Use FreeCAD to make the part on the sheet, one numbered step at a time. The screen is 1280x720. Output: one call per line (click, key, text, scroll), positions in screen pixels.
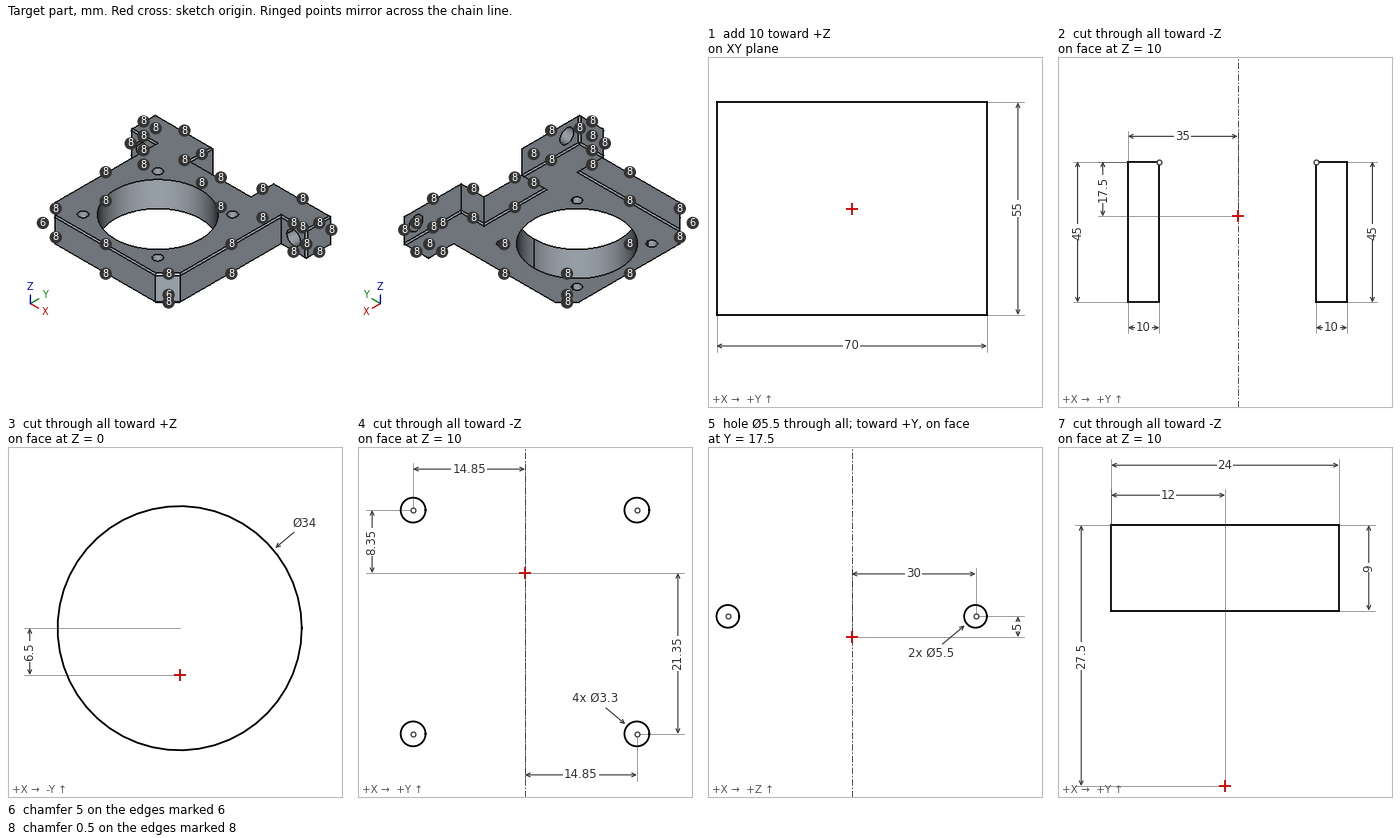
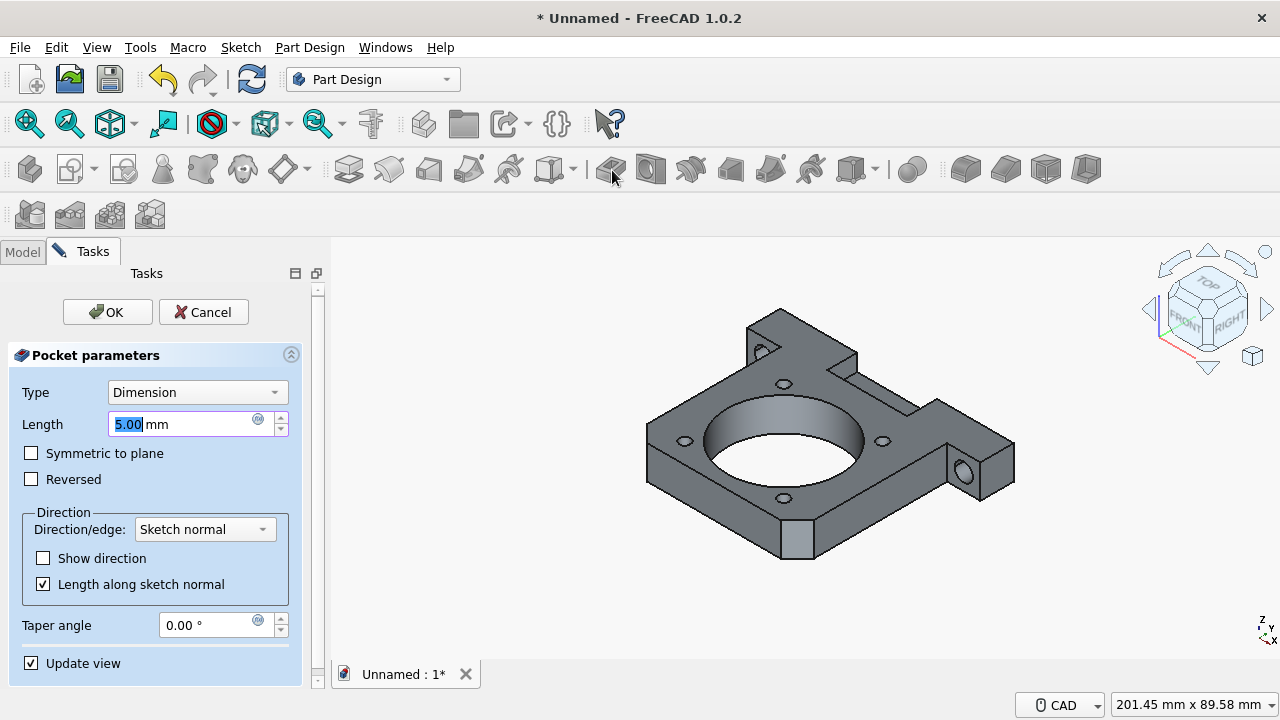
click(198, 392)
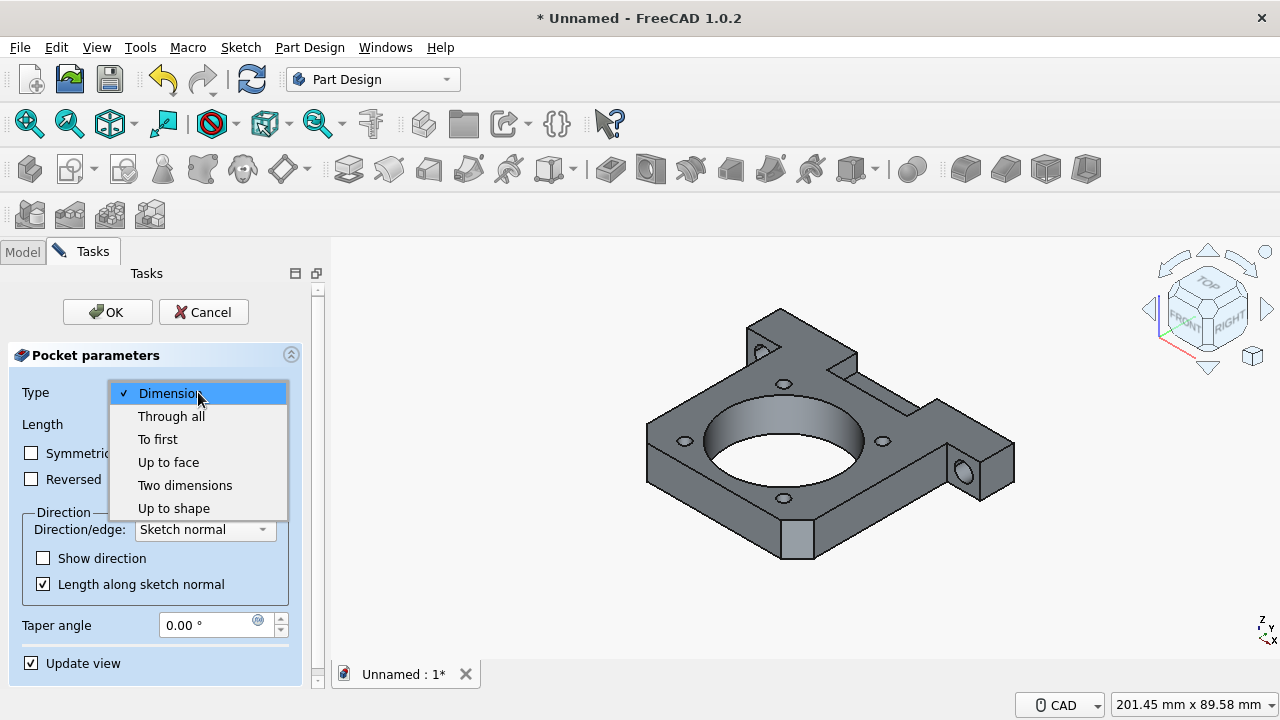
click(198, 416)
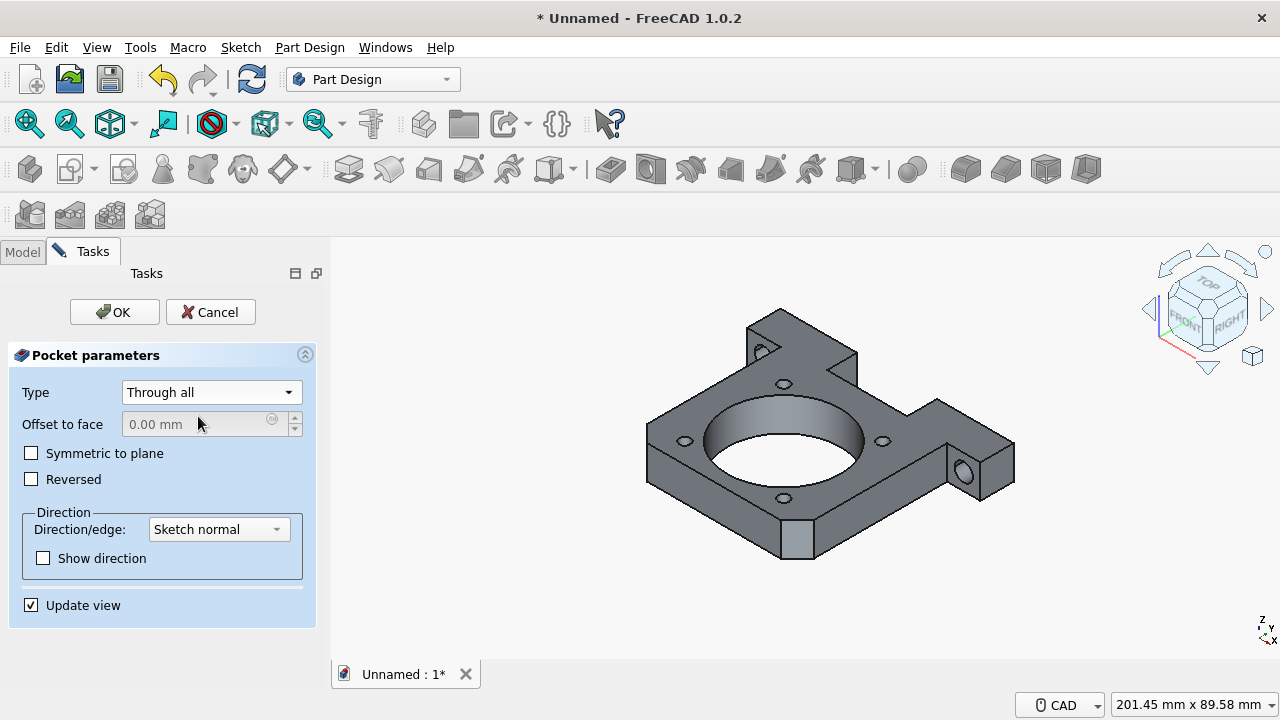
click(115, 312)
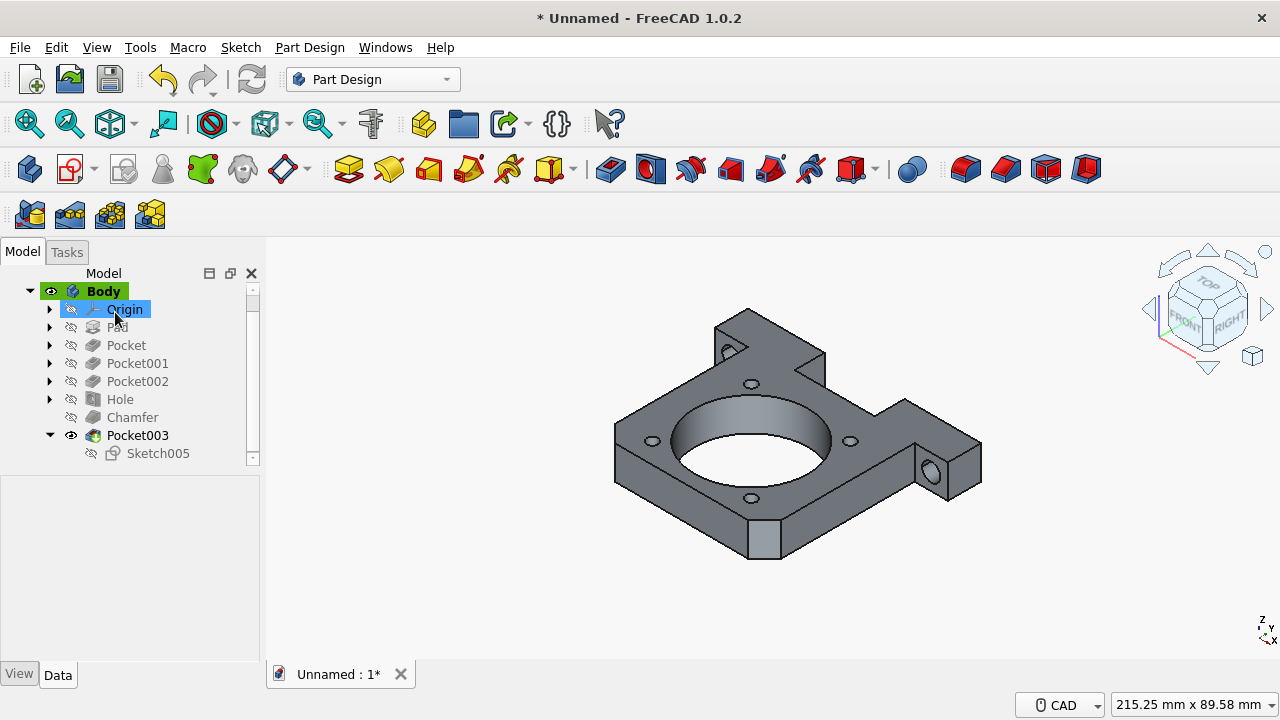
click(965, 471)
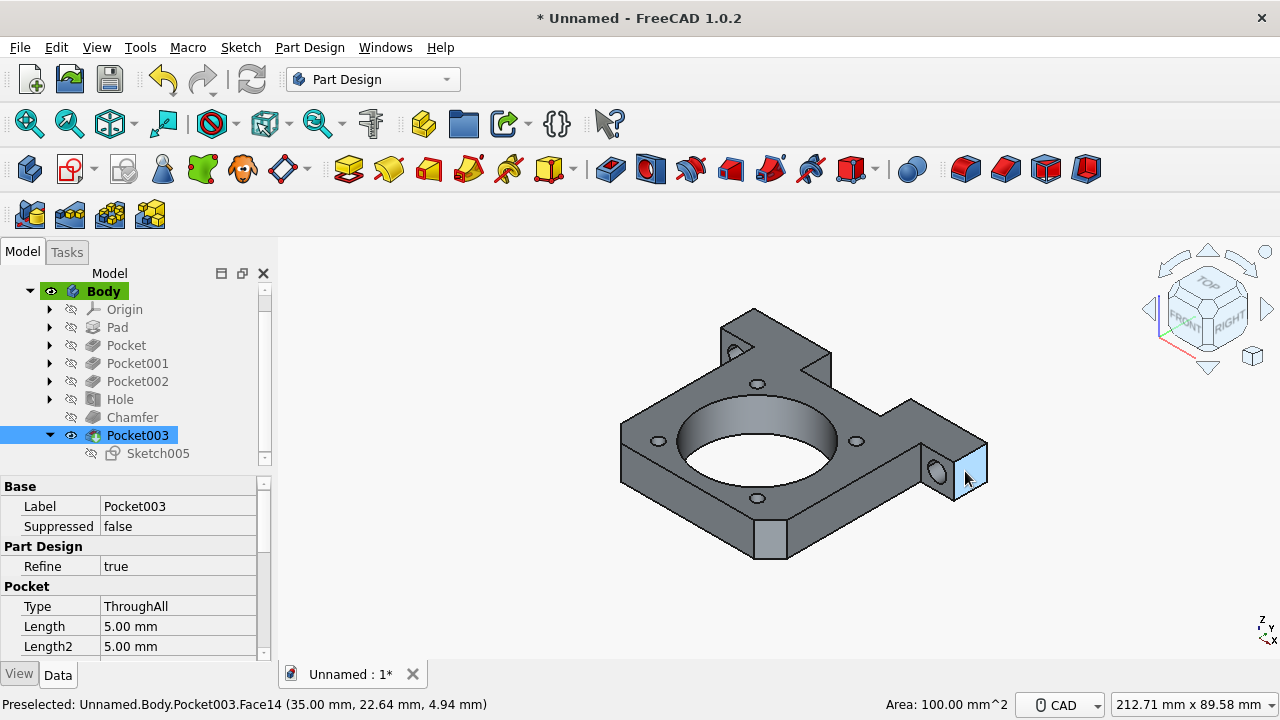
click(737, 336, ctrl)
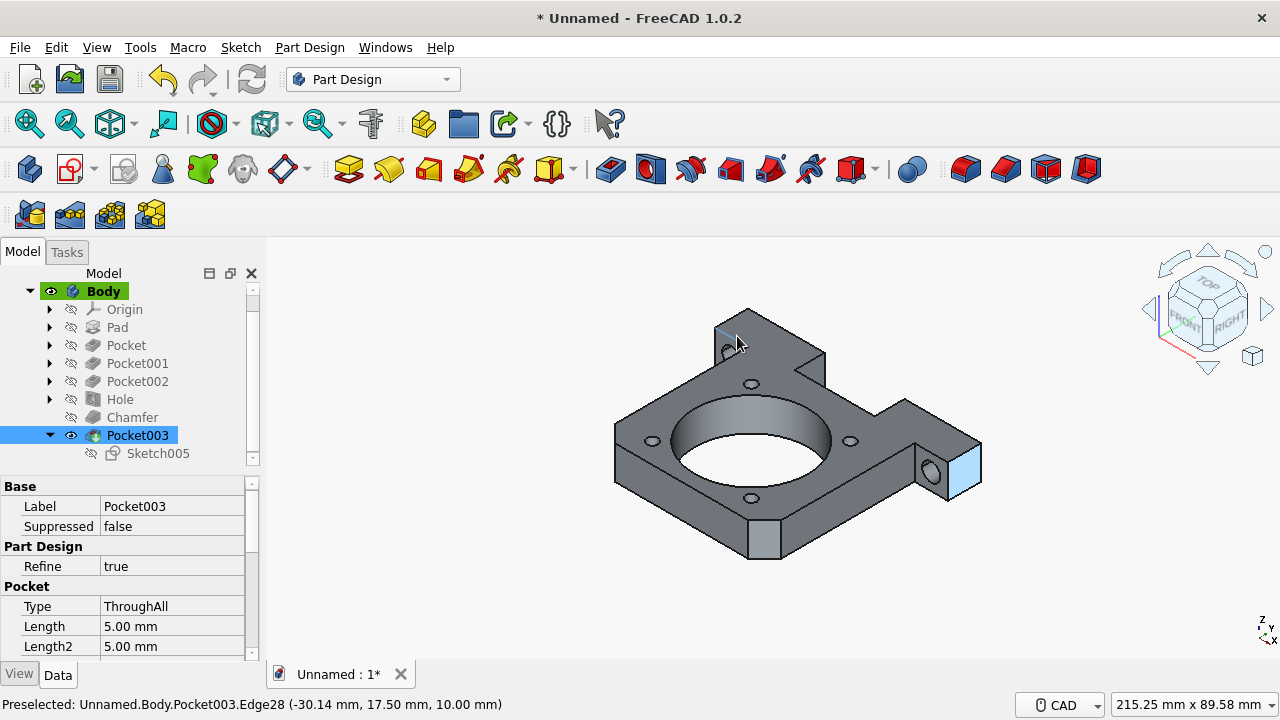
click(931, 452, ctrl)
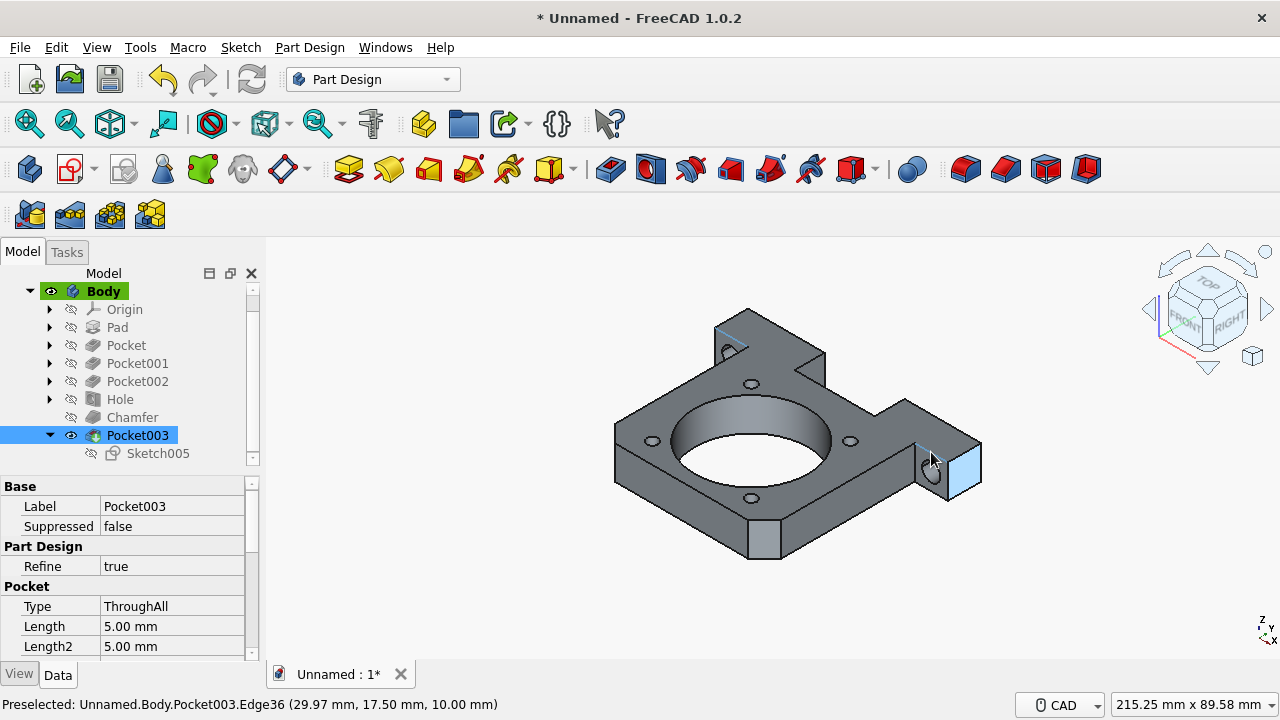
click(848, 481, ctrl)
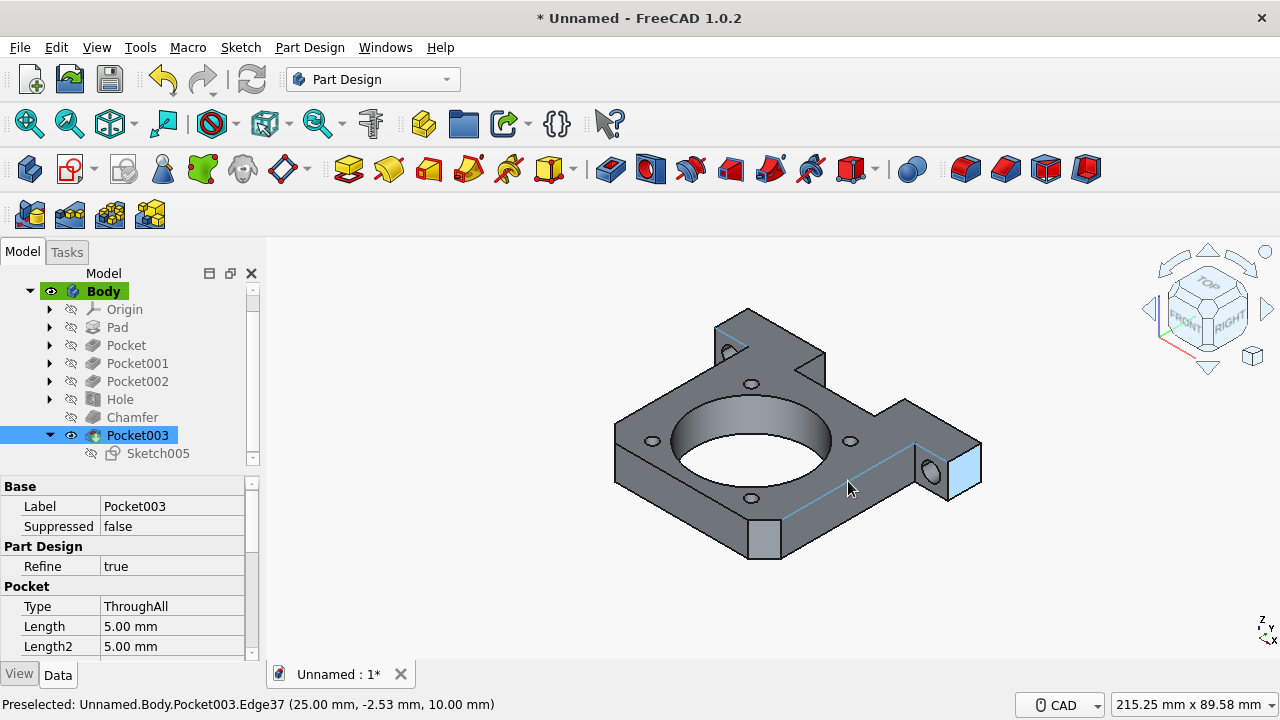
click(681, 481, ctrl)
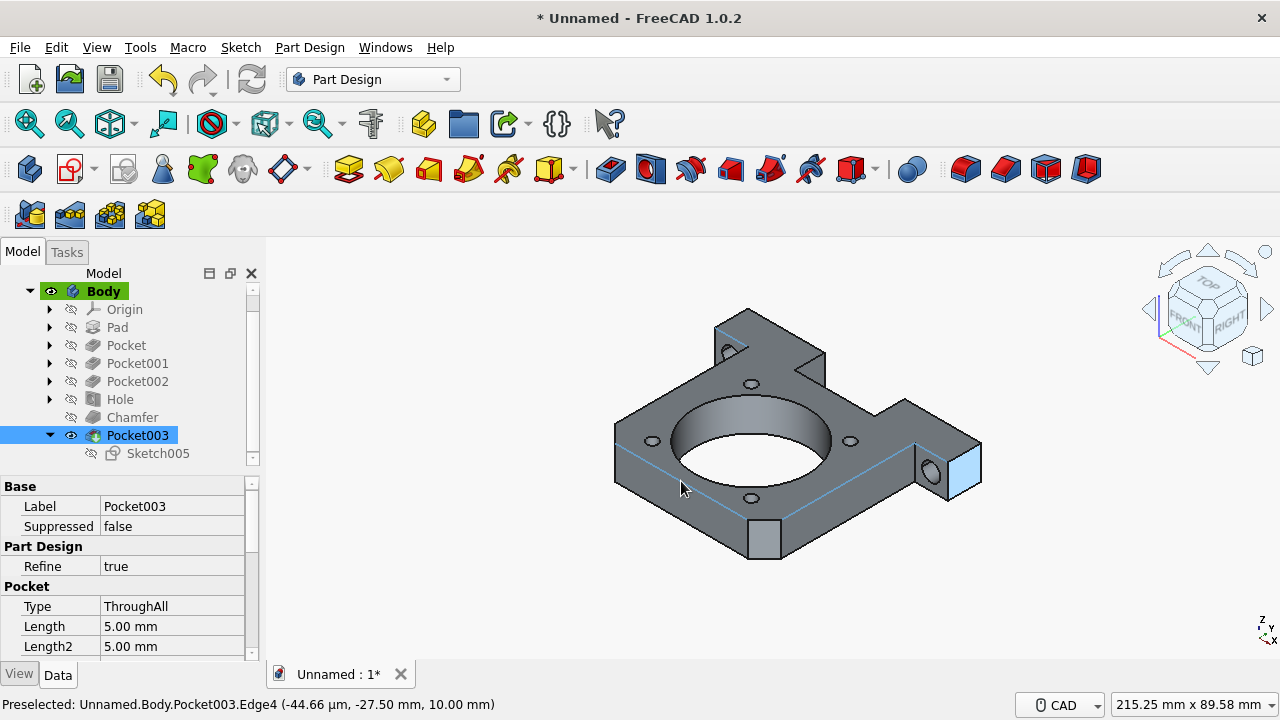
click(765, 519, ctrl)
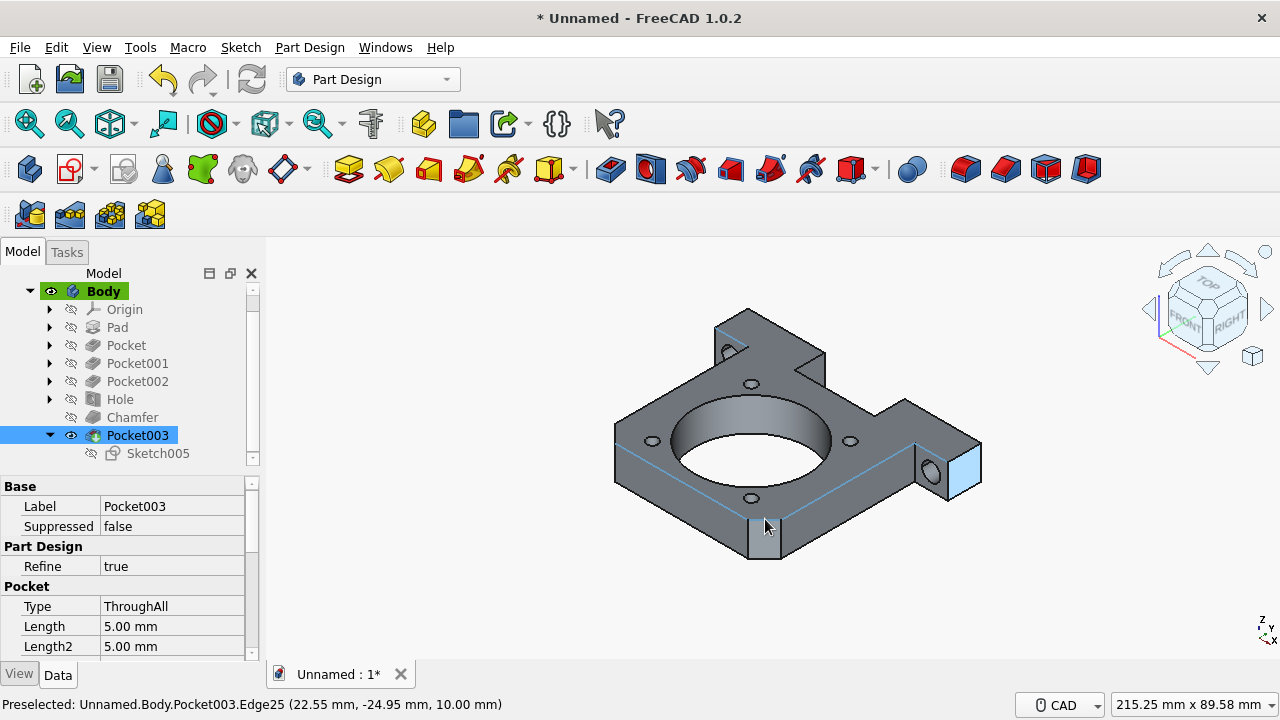
click(810, 360, ctrl)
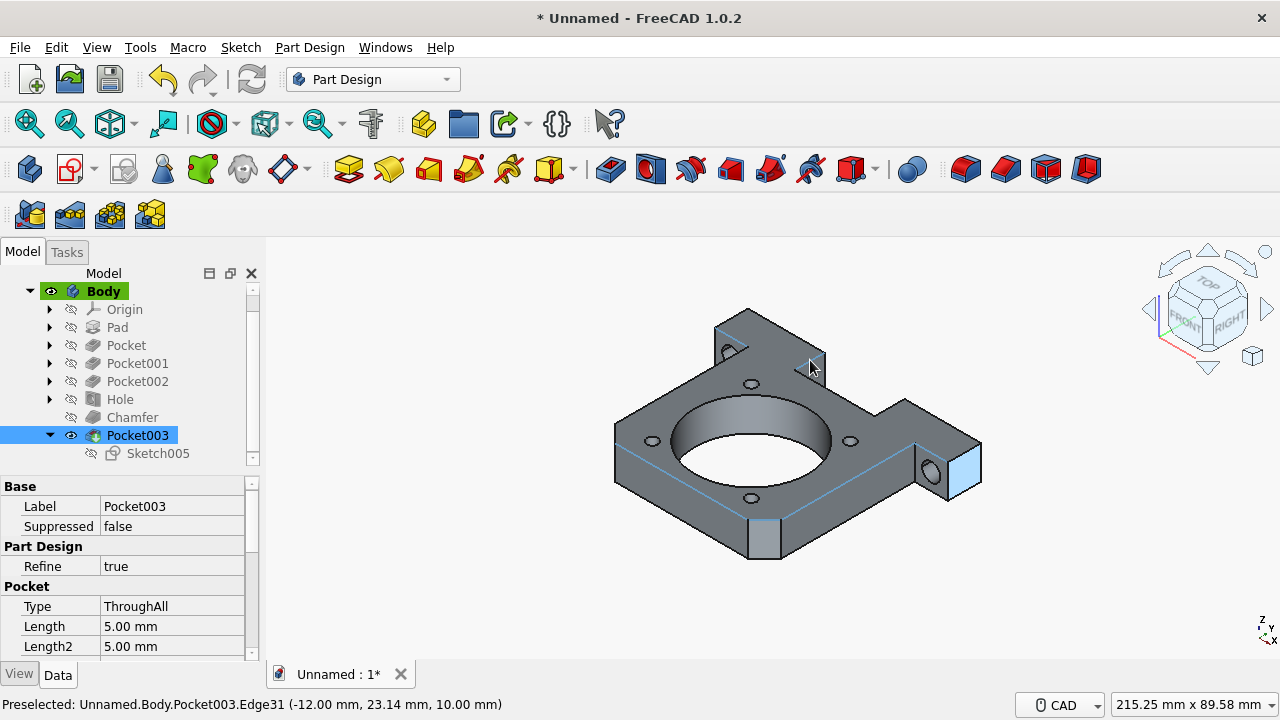
key(2)